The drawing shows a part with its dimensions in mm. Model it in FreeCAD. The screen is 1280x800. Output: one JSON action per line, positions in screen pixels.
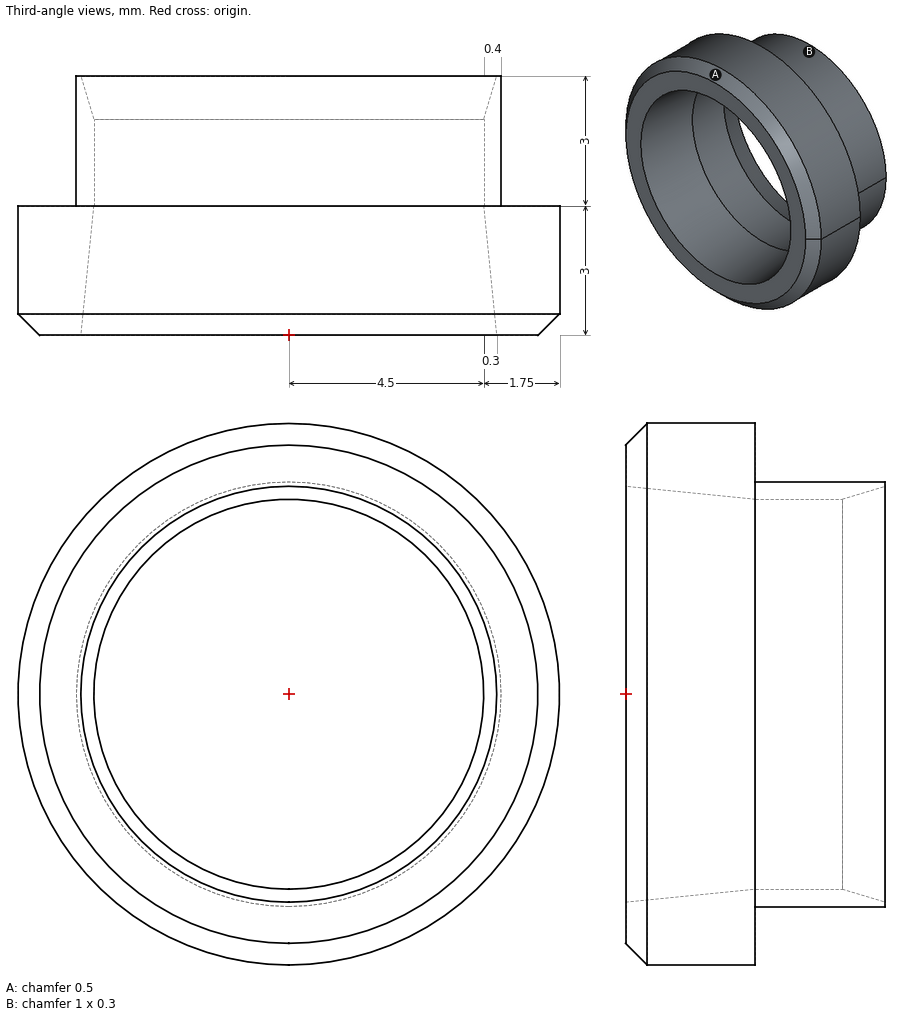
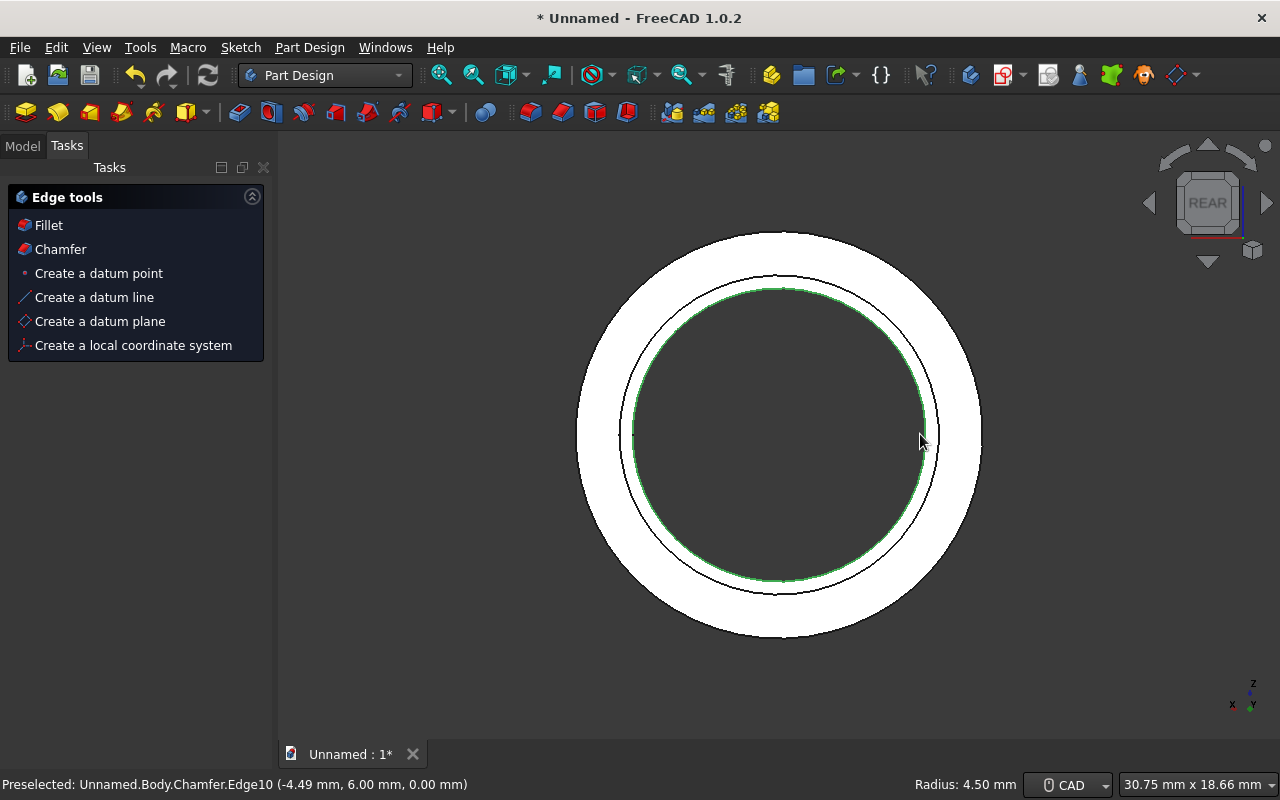
{"action": "left_click", "coordinate": [564, 112]}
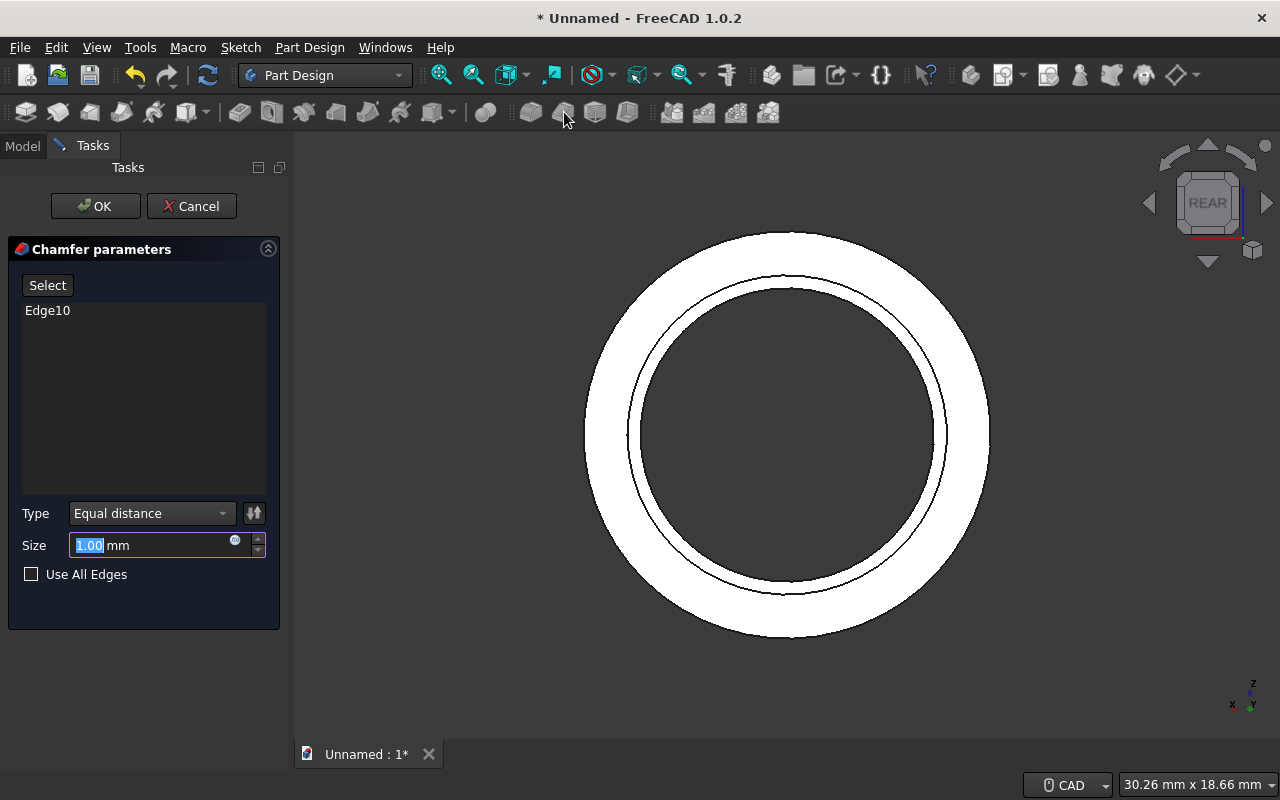
{"action": "type", "text": "1"}
{"action": "key", "text": "Tab"}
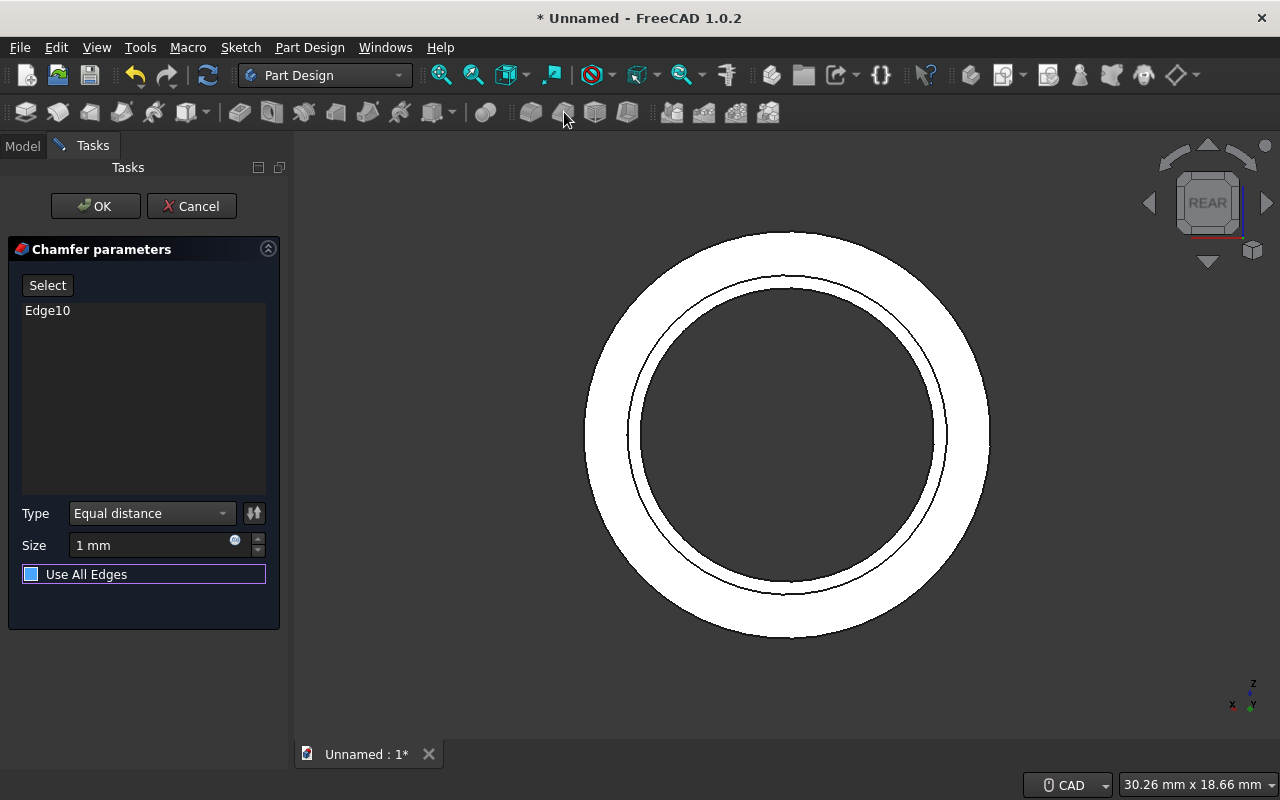
{"action": "left_click", "coordinate": [153, 514]}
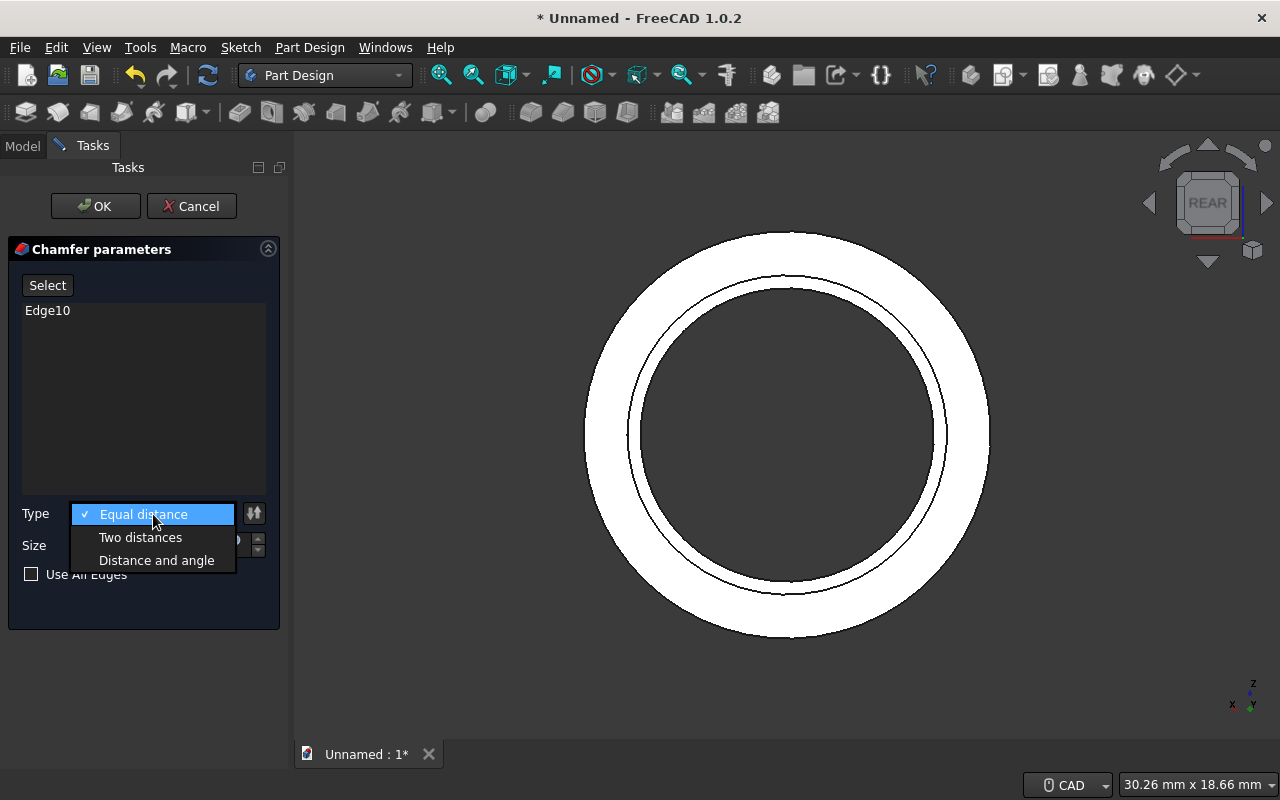
{"action": "left_click", "coordinate": [152, 538]}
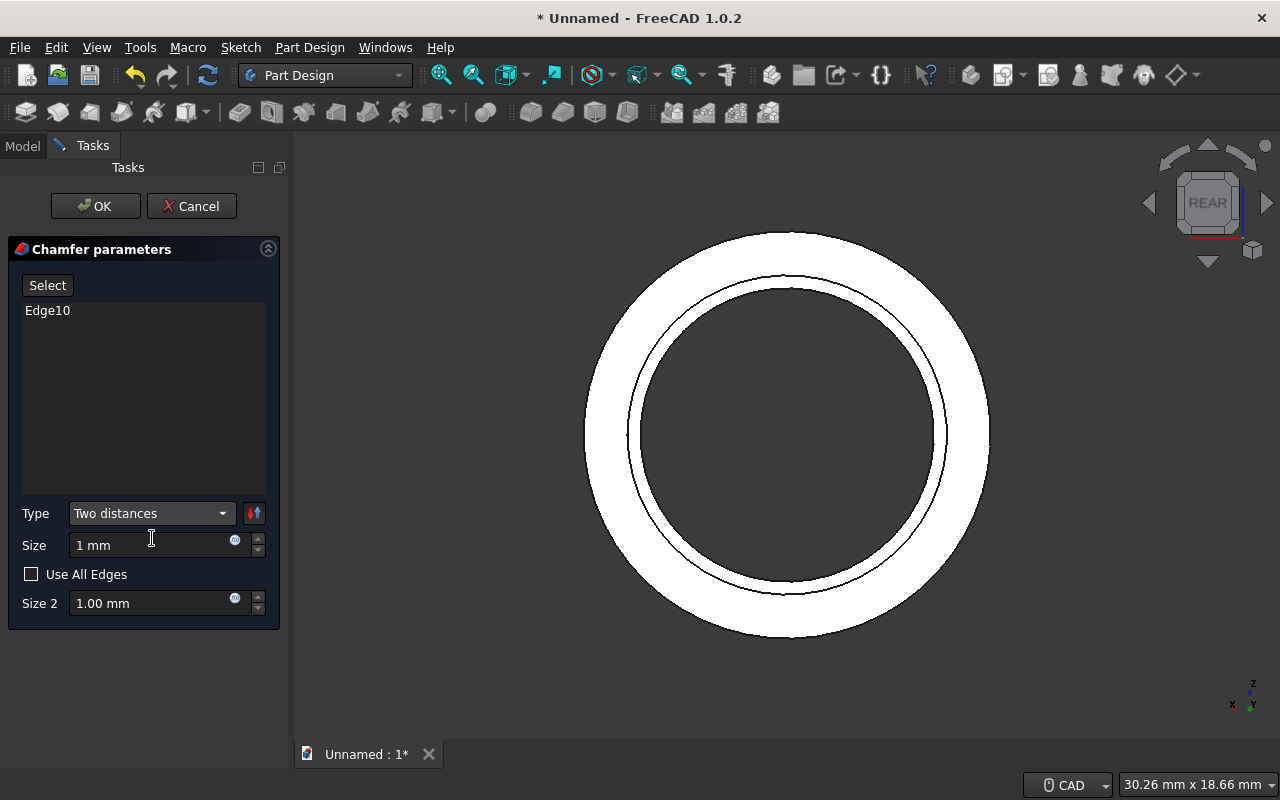
{"action": "triple_click", "coordinate": [160, 603]}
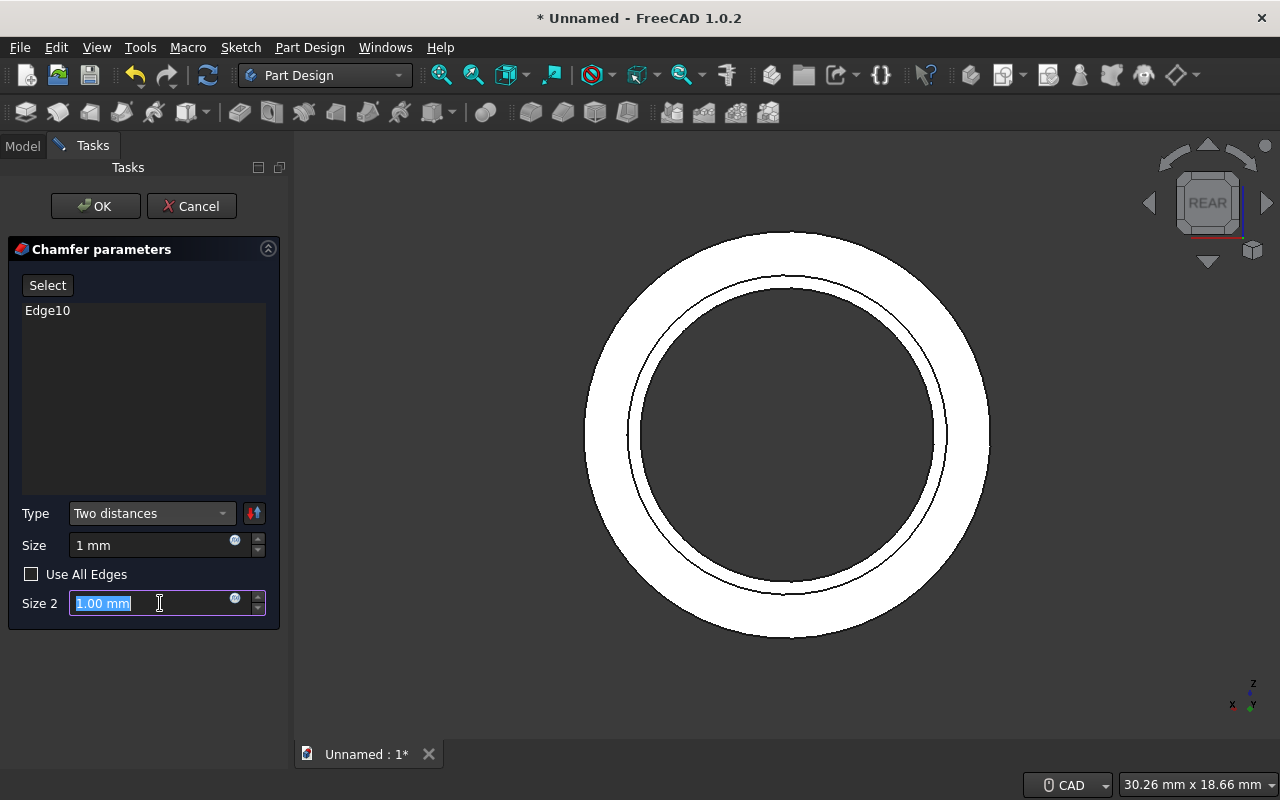
{"action": "type", "text": "0.3"}
{"action": "key", "text": "Tab"}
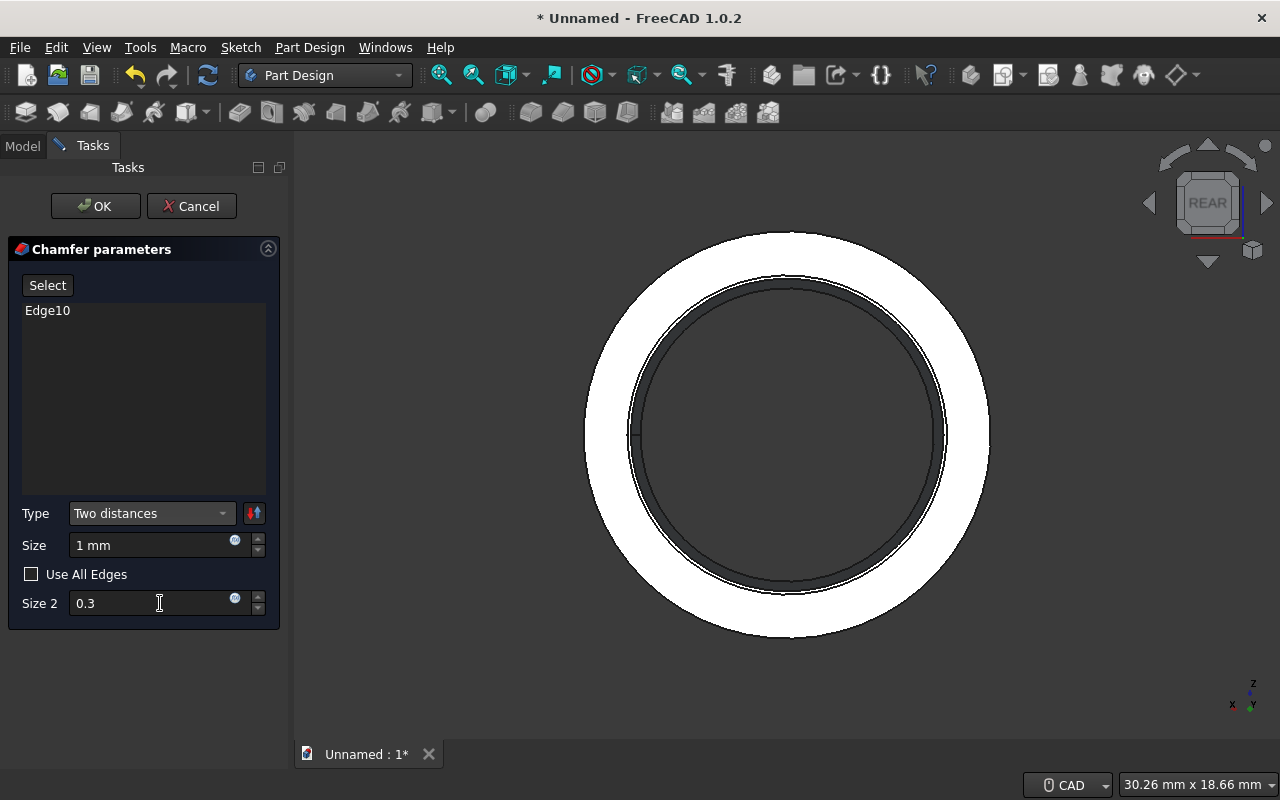
{"action": "left_click", "coordinate": [96, 206]}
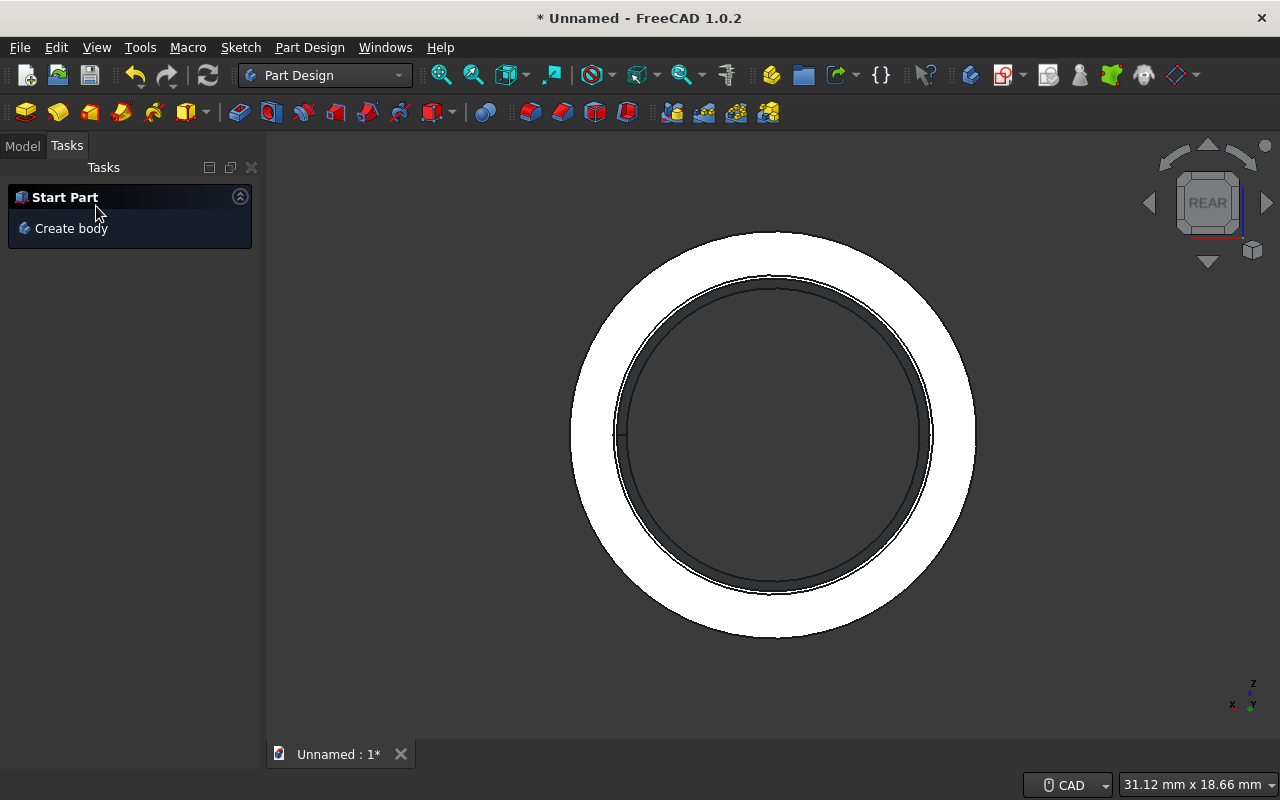
{"action": "key", "text": "0"}